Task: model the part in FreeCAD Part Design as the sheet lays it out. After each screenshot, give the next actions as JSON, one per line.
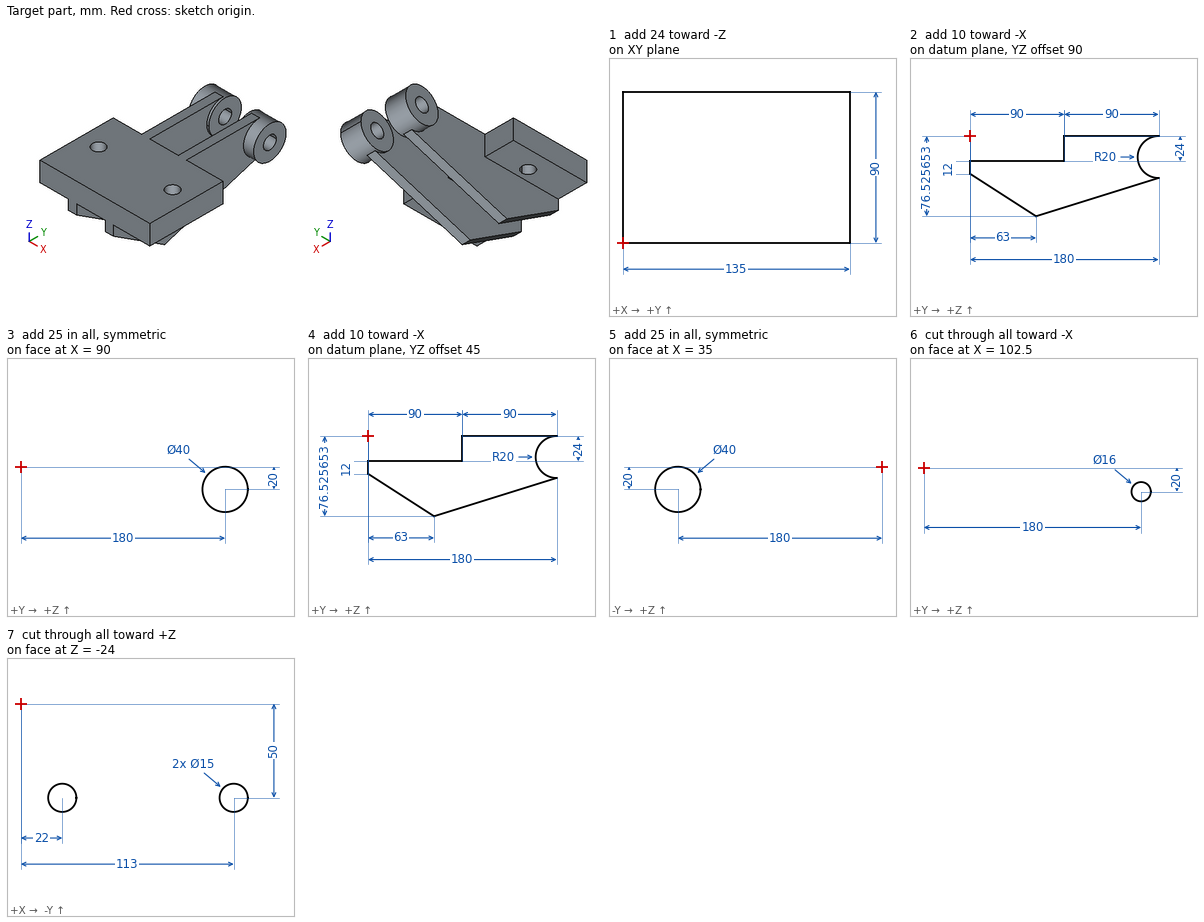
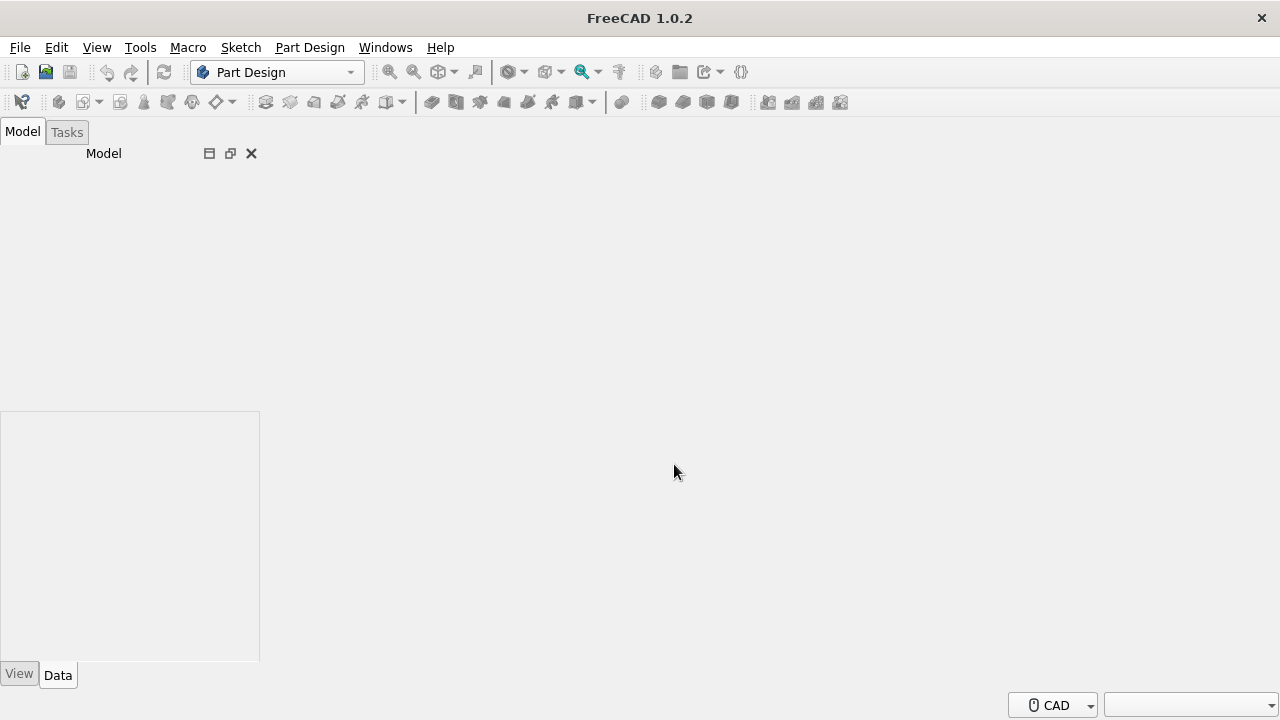
{"action": "left_click", "coordinate": [22, 72]}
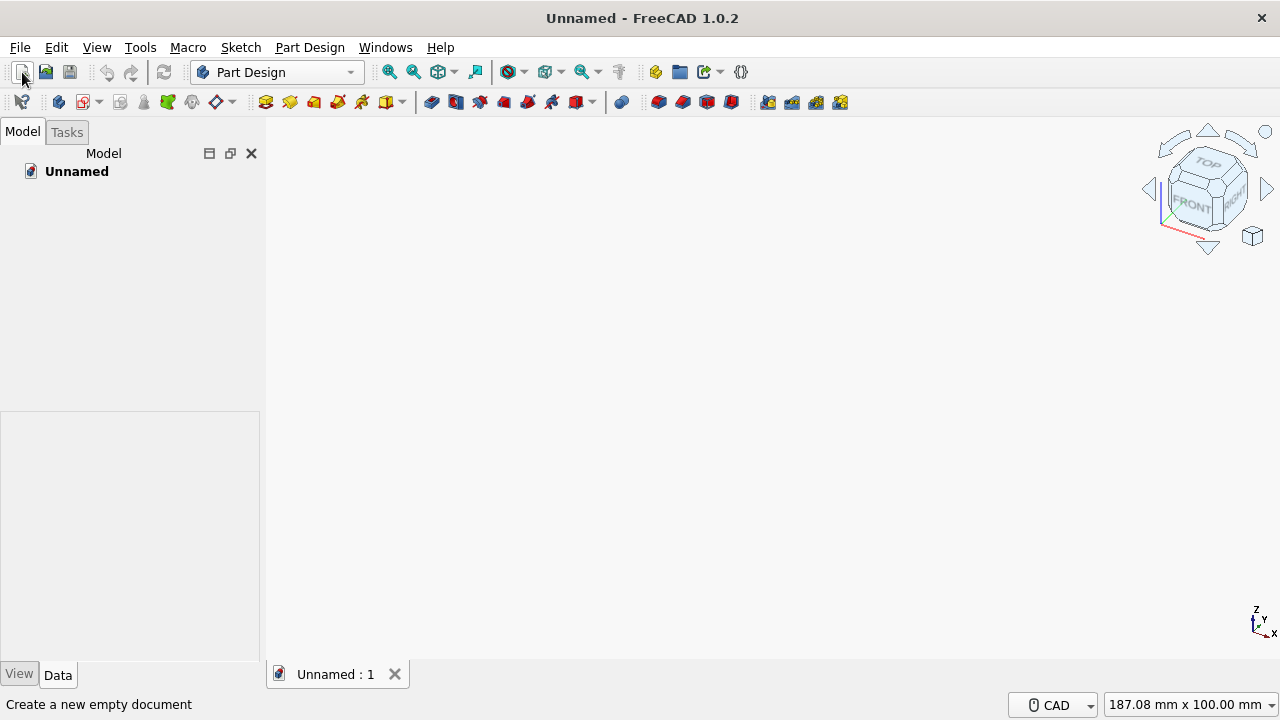
{"action": "left_click", "coordinate": [84, 102]}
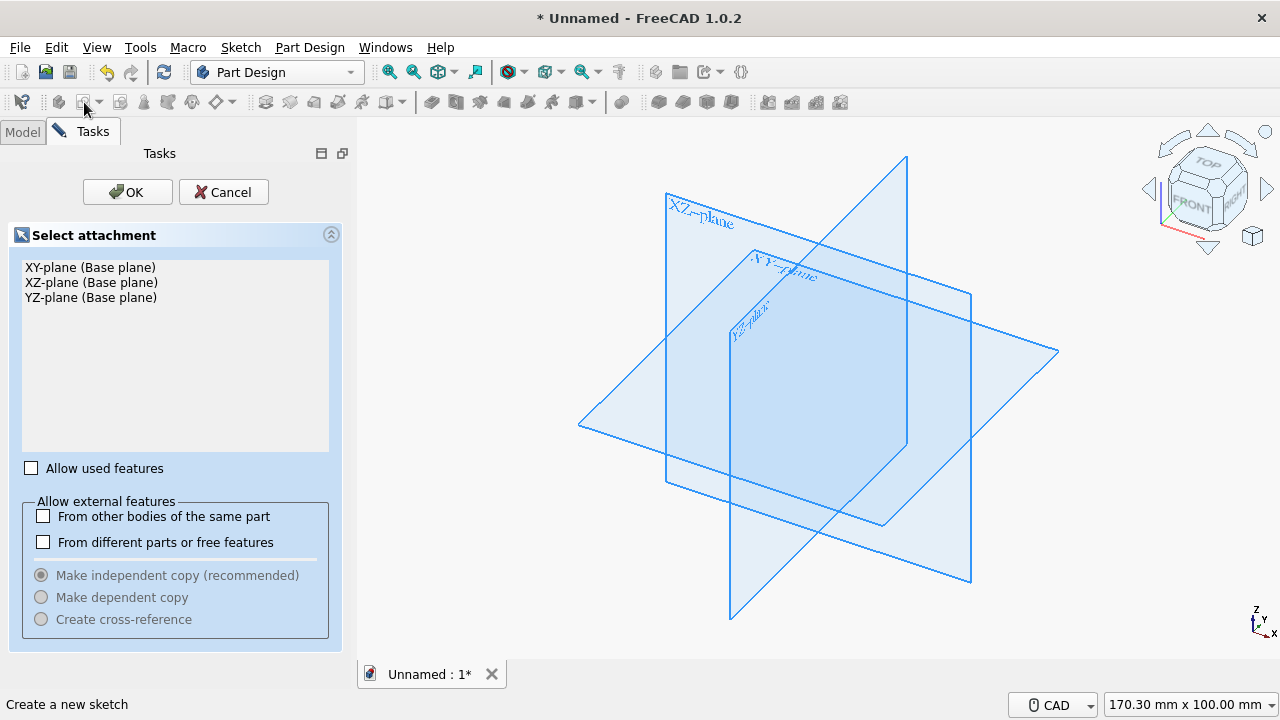
{"action": "left_click", "coordinate": [82, 268]}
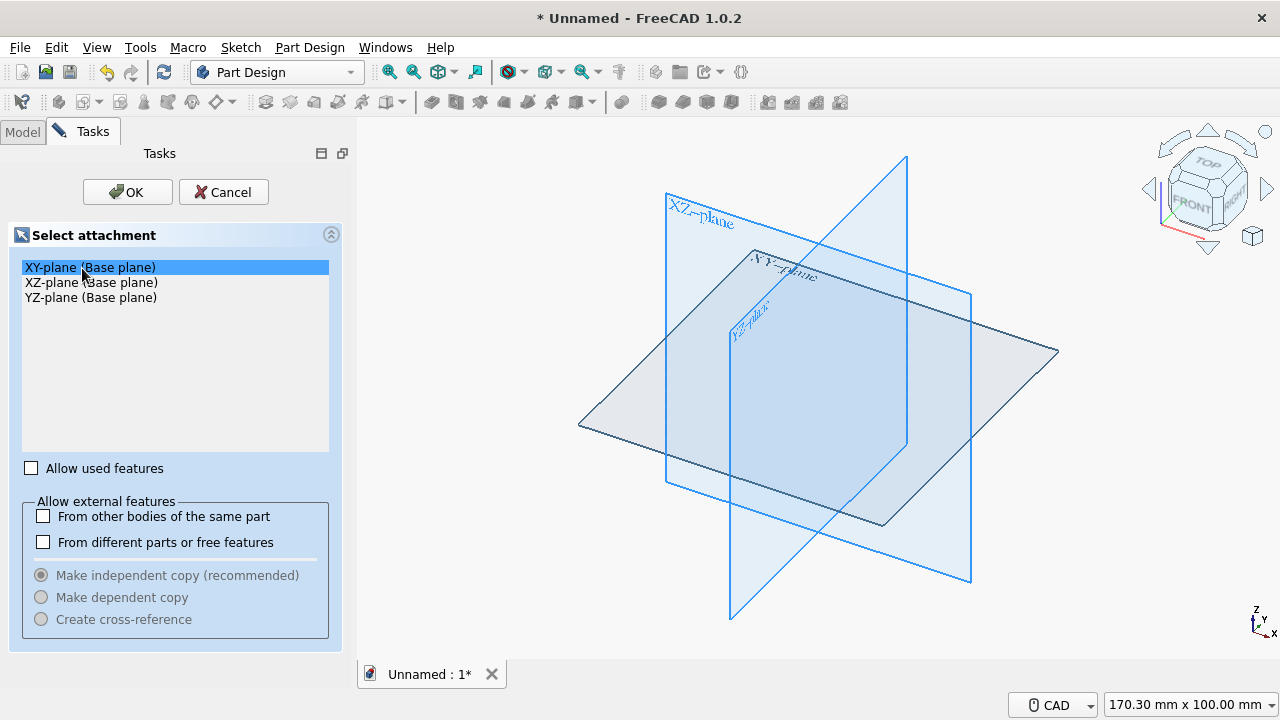
{"action": "left_click", "coordinate": [128, 192]}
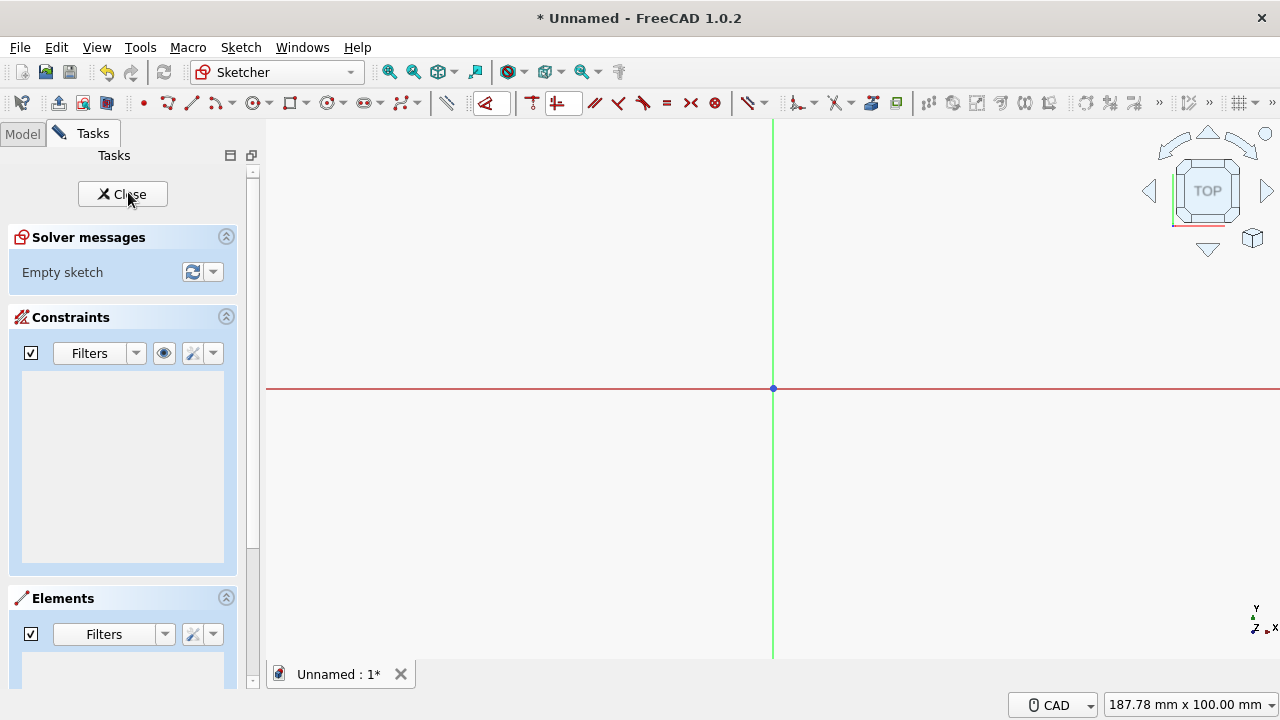
{"action": "scroll", "coordinate": [294, 631], "scroll_direction": "down", "scroll_amount": 3}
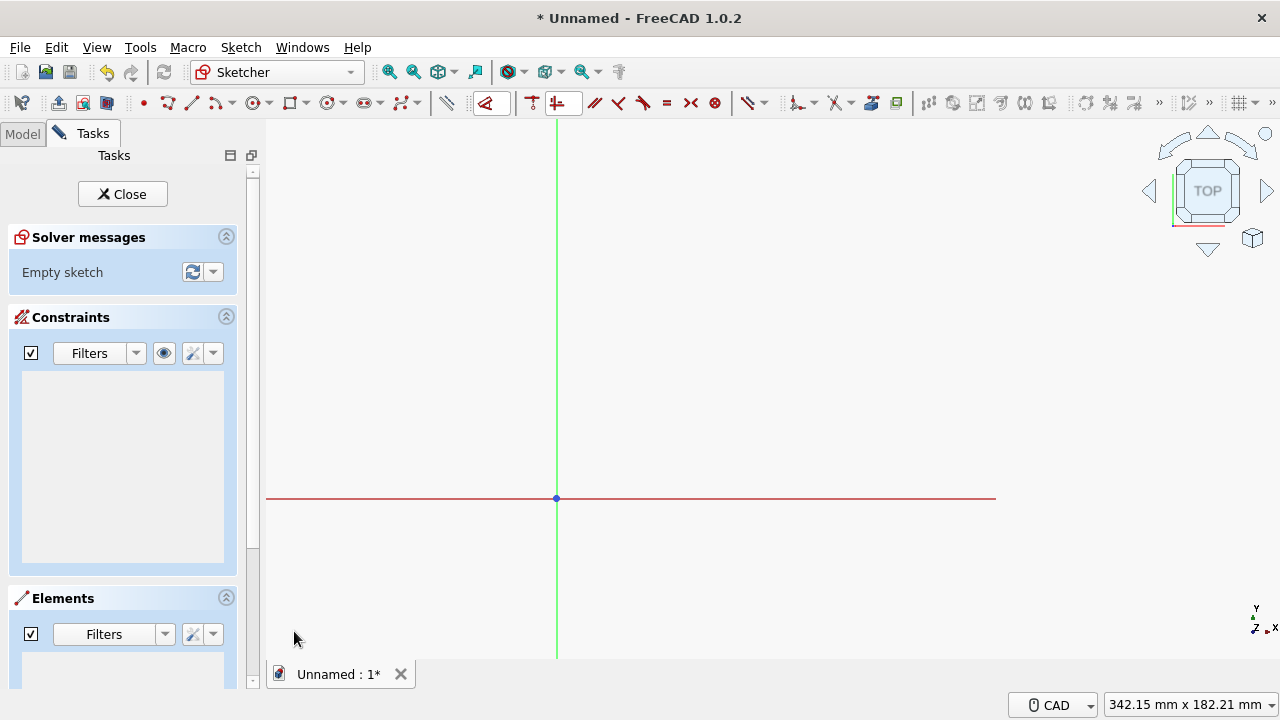
{"action": "key", "text": "g r"}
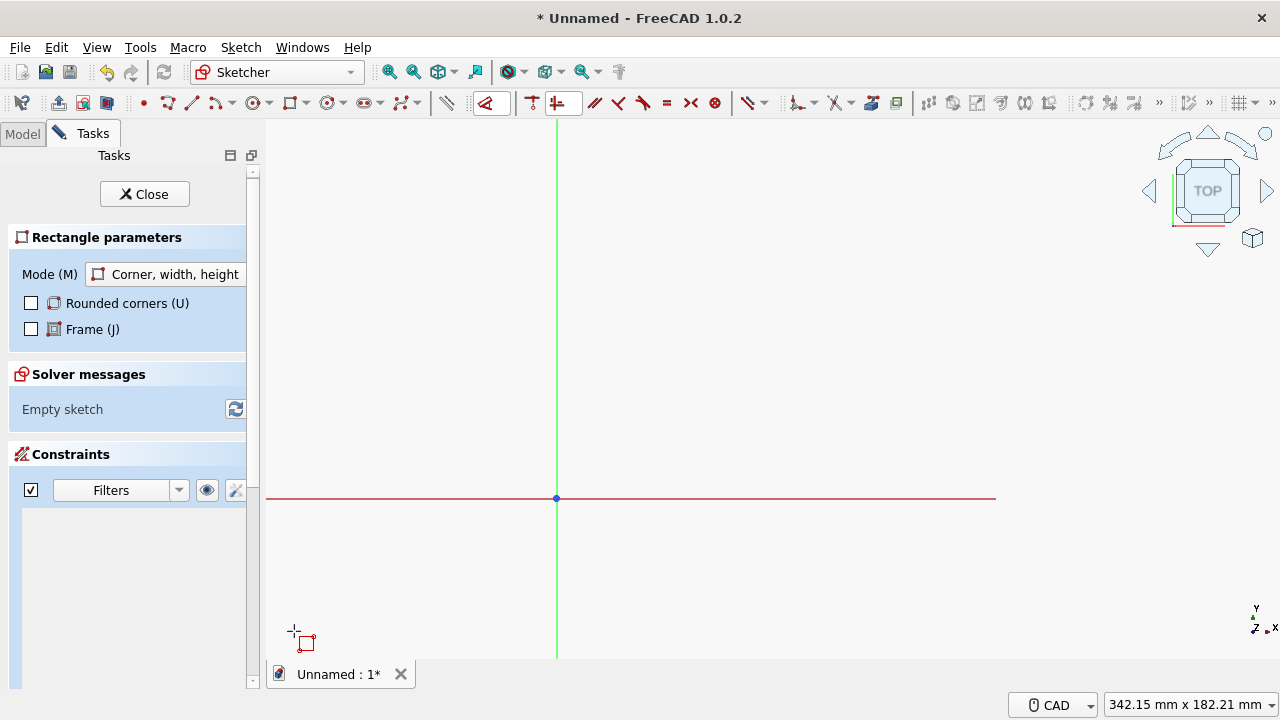
{"action": "left_click", "coordinate": [557, 499]}
{"action": "mouse_move", "coordinate": [957, 232]}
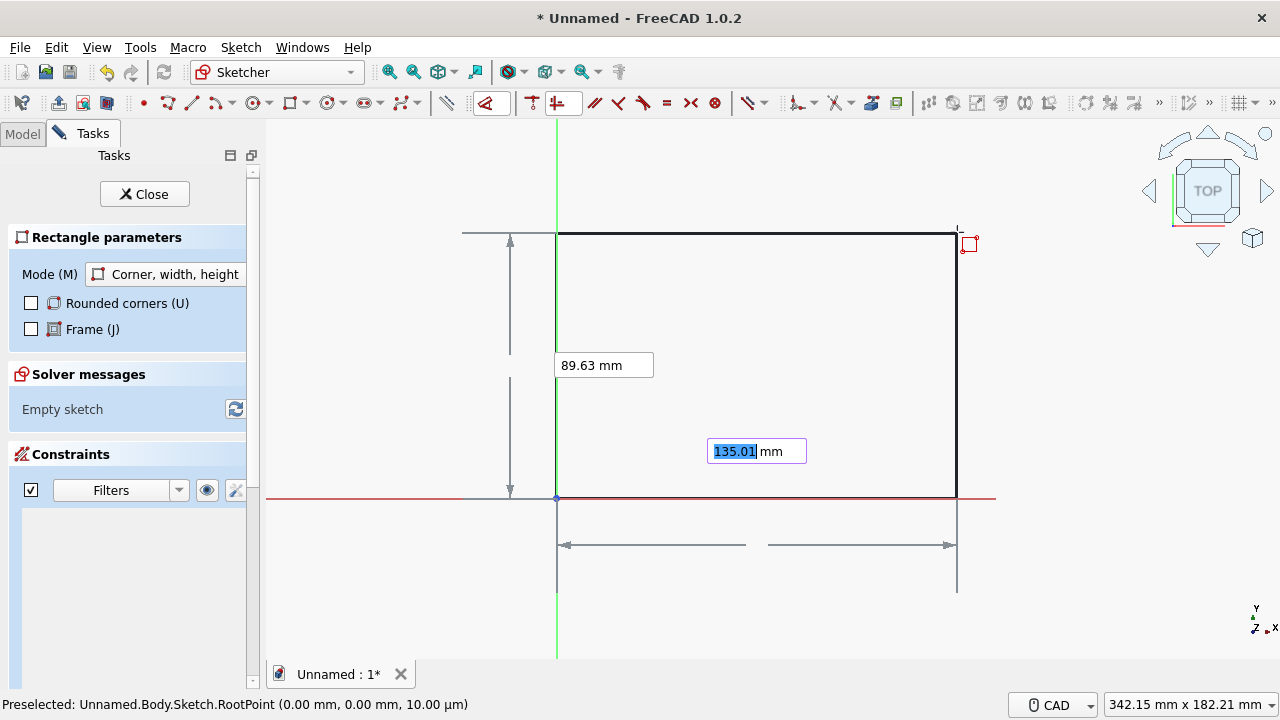
{"action": "type", "text": "135"}
{"action": "key", "text": "Tab"}
{"action": "type", "text": "90"}
{"action": "key", "text": "Return"}
{"action": "key", "text": "Escape"}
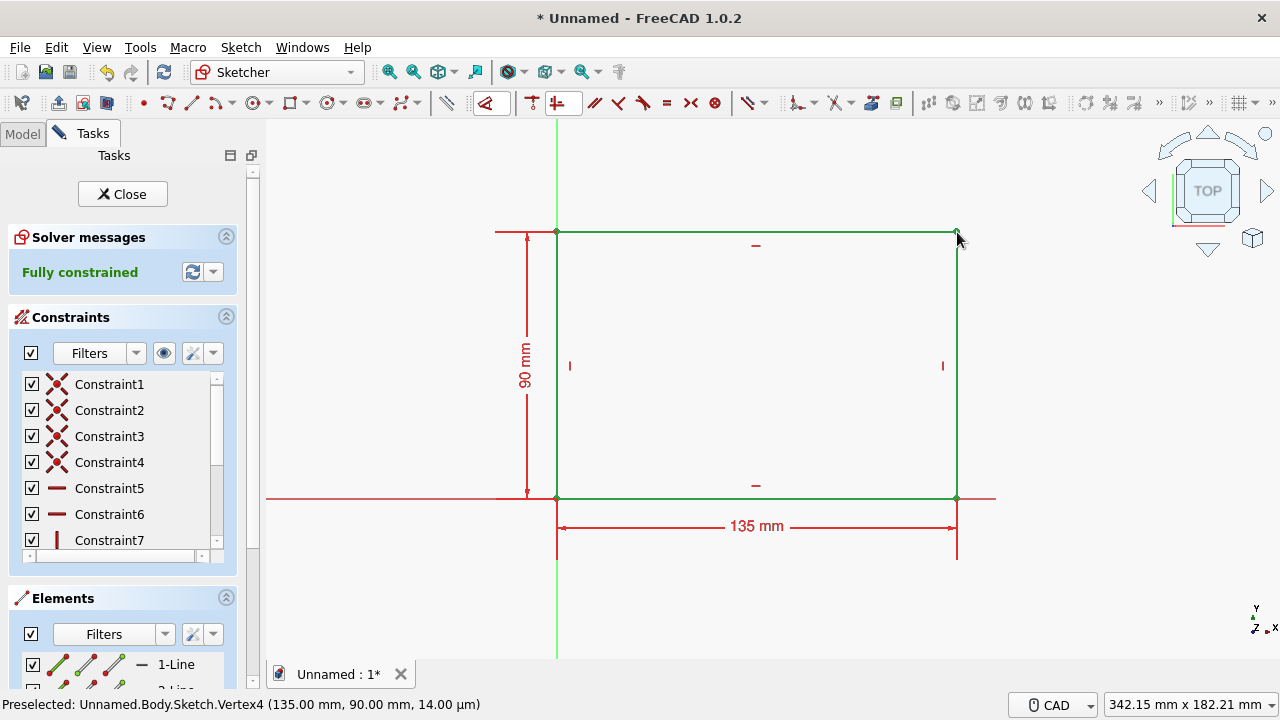
{"action": "left_click", "coordinate": [123, 194]}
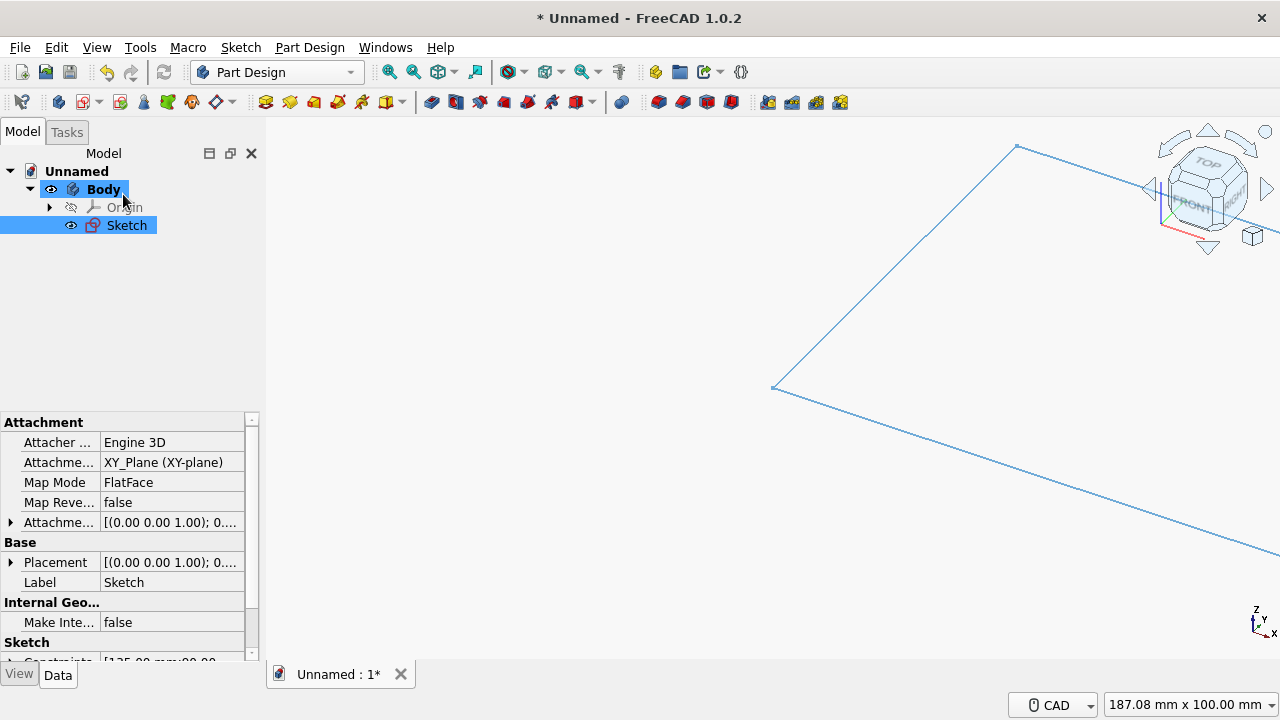
{"action": "left_click", "coordinate": [266, 102]}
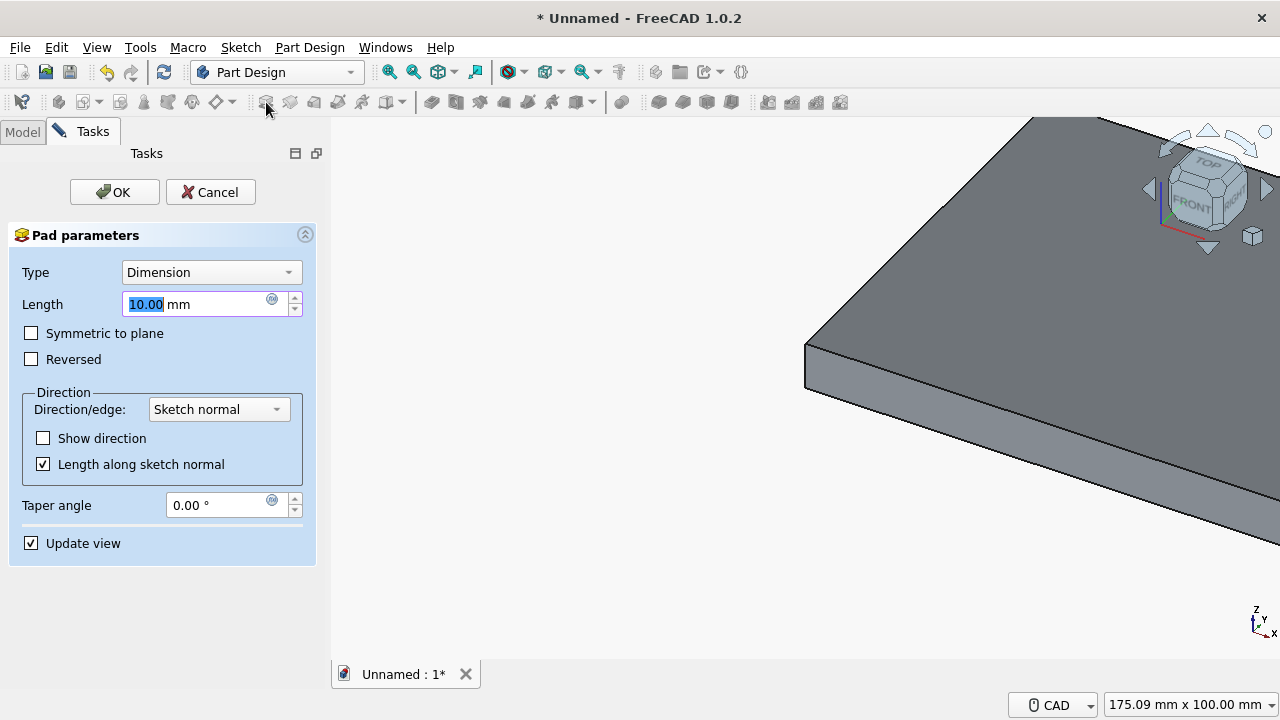
{"action": "type", "text": "24"}
{"action": "key", "text": "Tab"}